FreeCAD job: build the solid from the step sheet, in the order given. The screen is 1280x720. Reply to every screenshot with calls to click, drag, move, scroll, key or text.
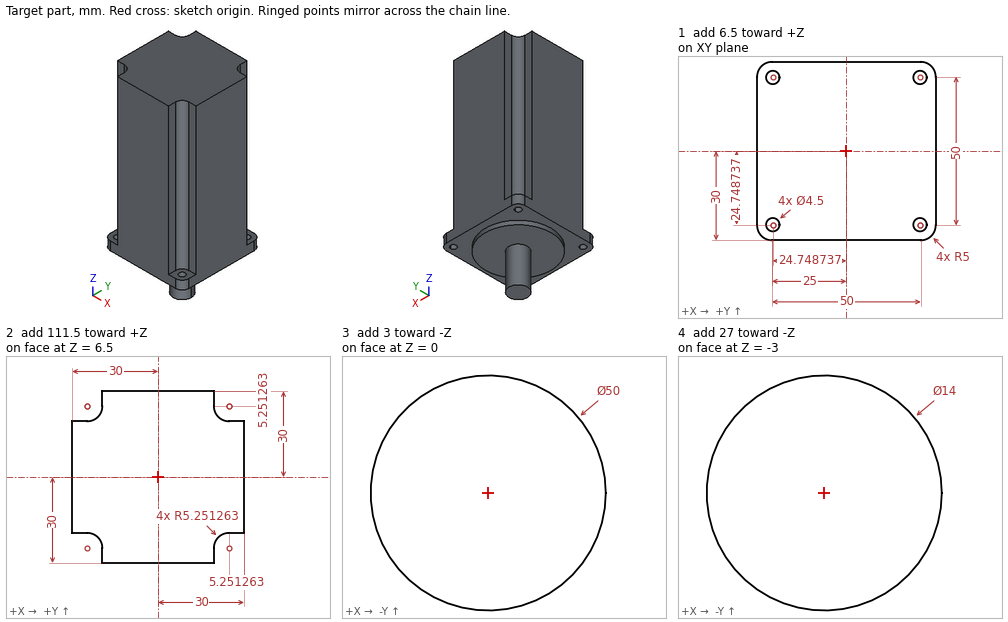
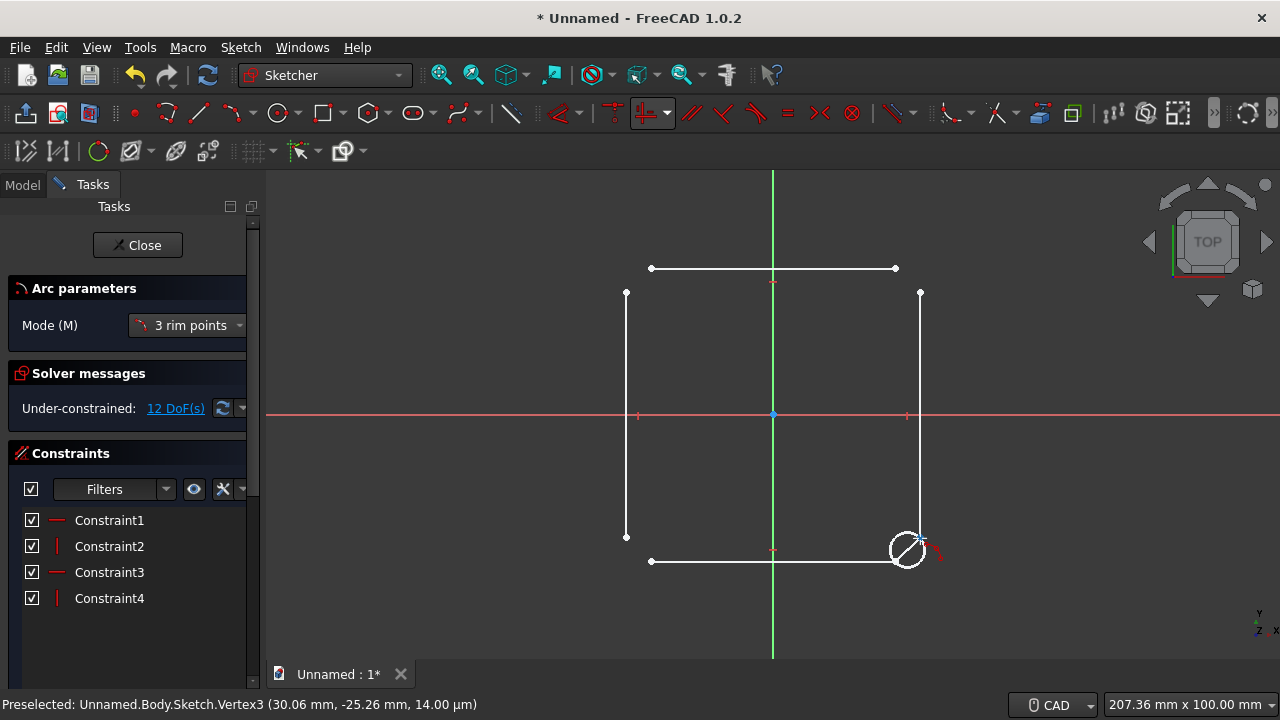
scroll(913, 554, up, 4)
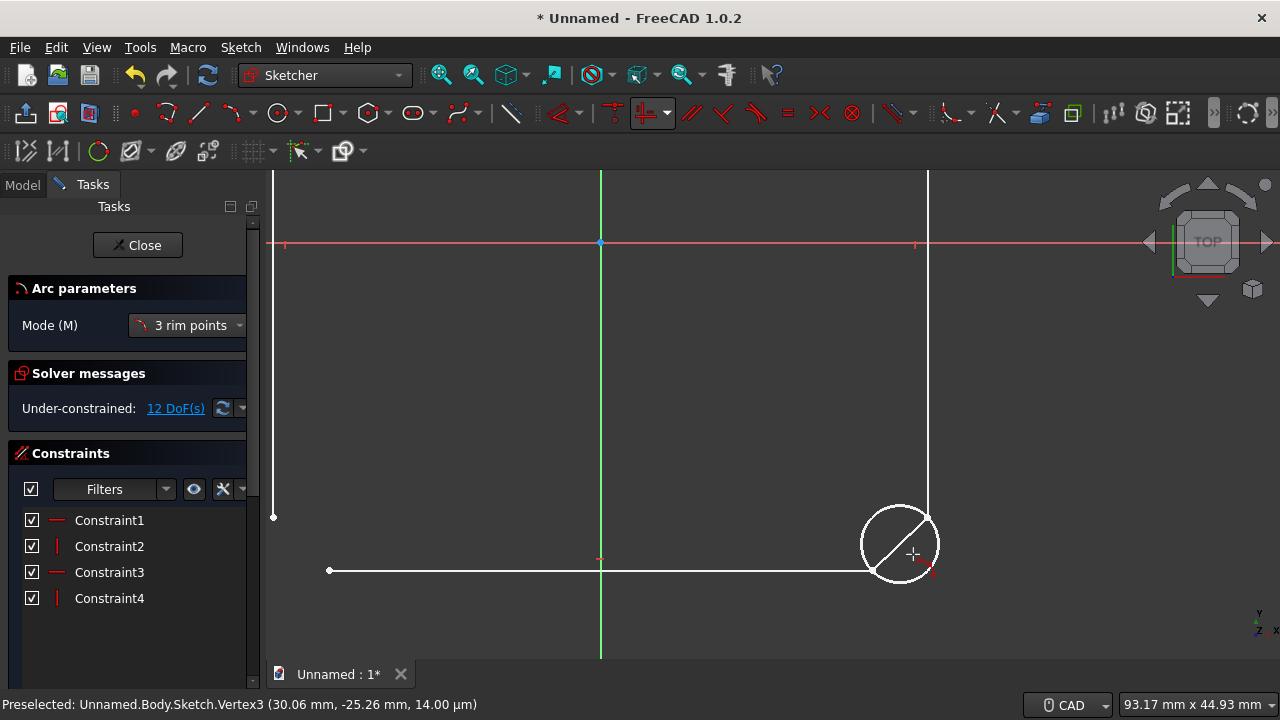
click(911, 553)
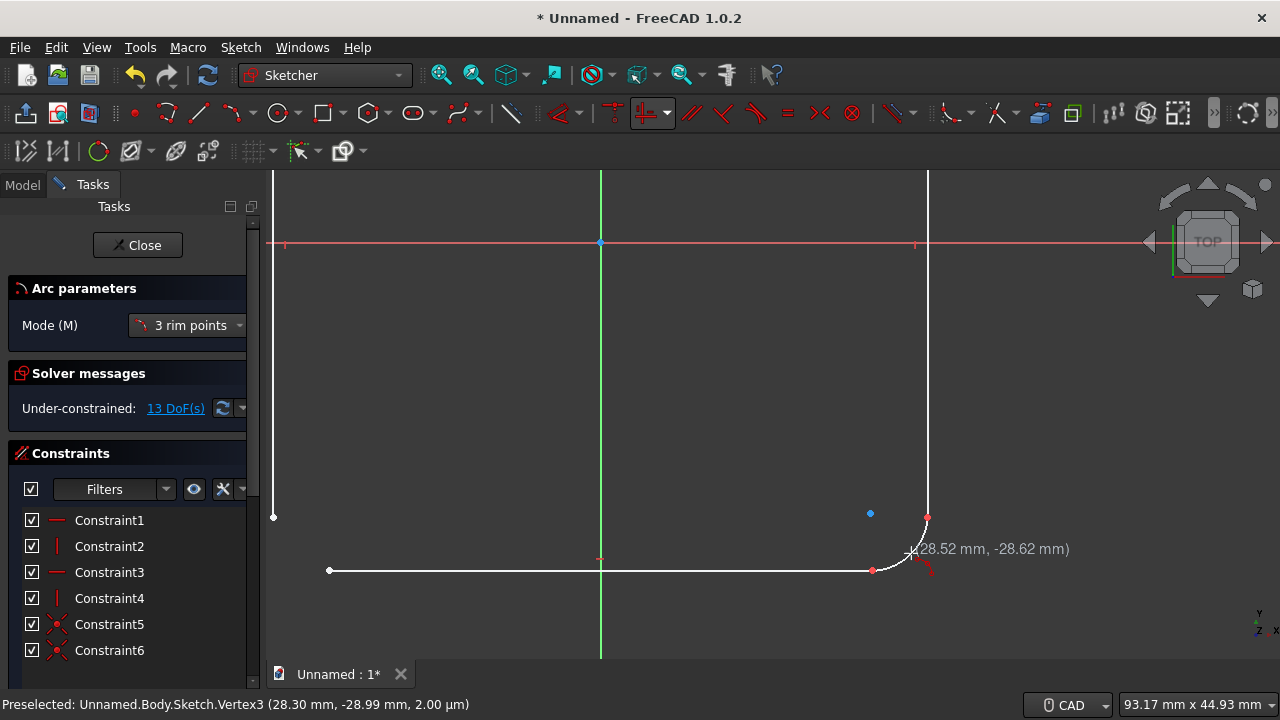
scroll(789, 555, down, 4)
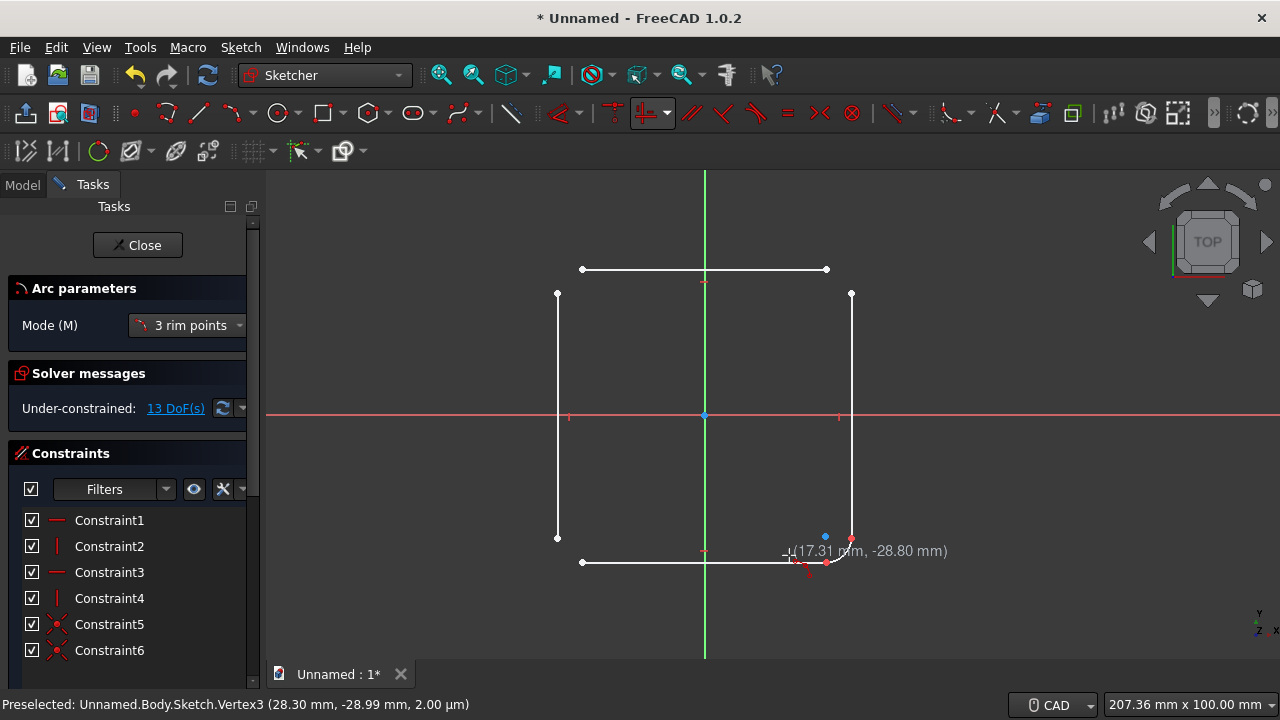
click(852, 294)
click(827, 270)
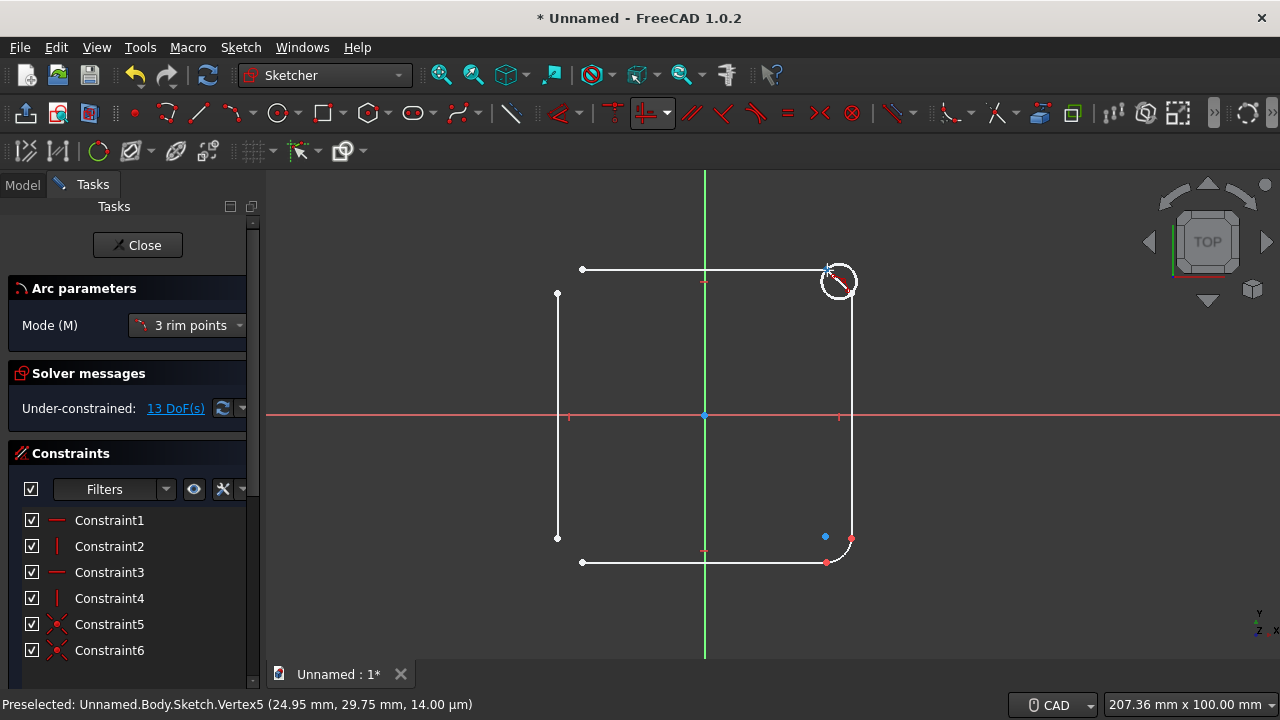
scroll(844, 276, up, 4)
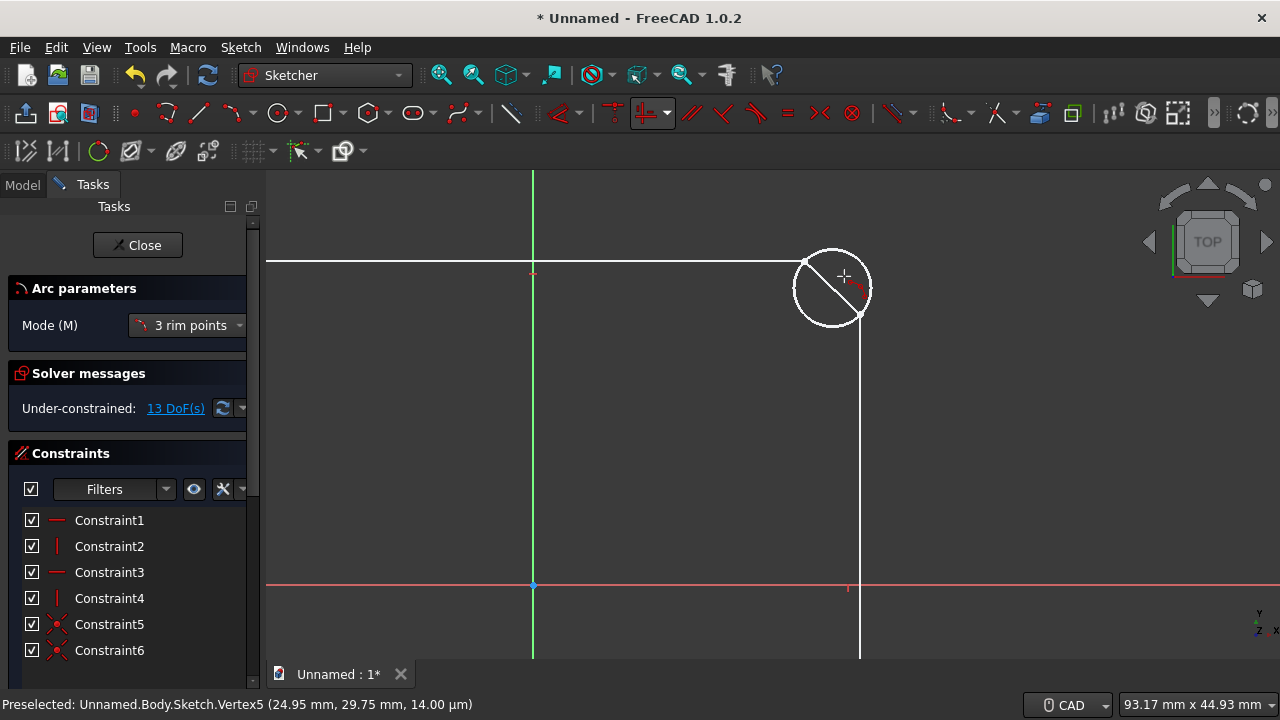
click(844, 275)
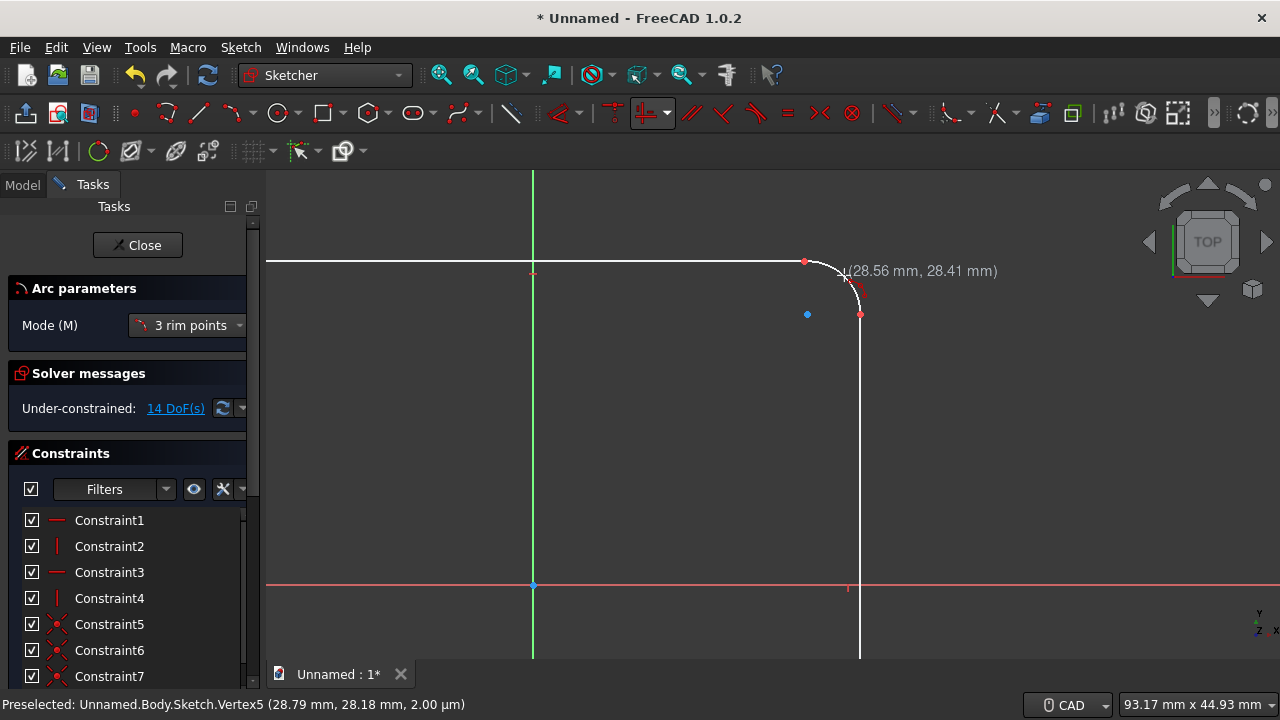
scroll(844, 275, down, 4)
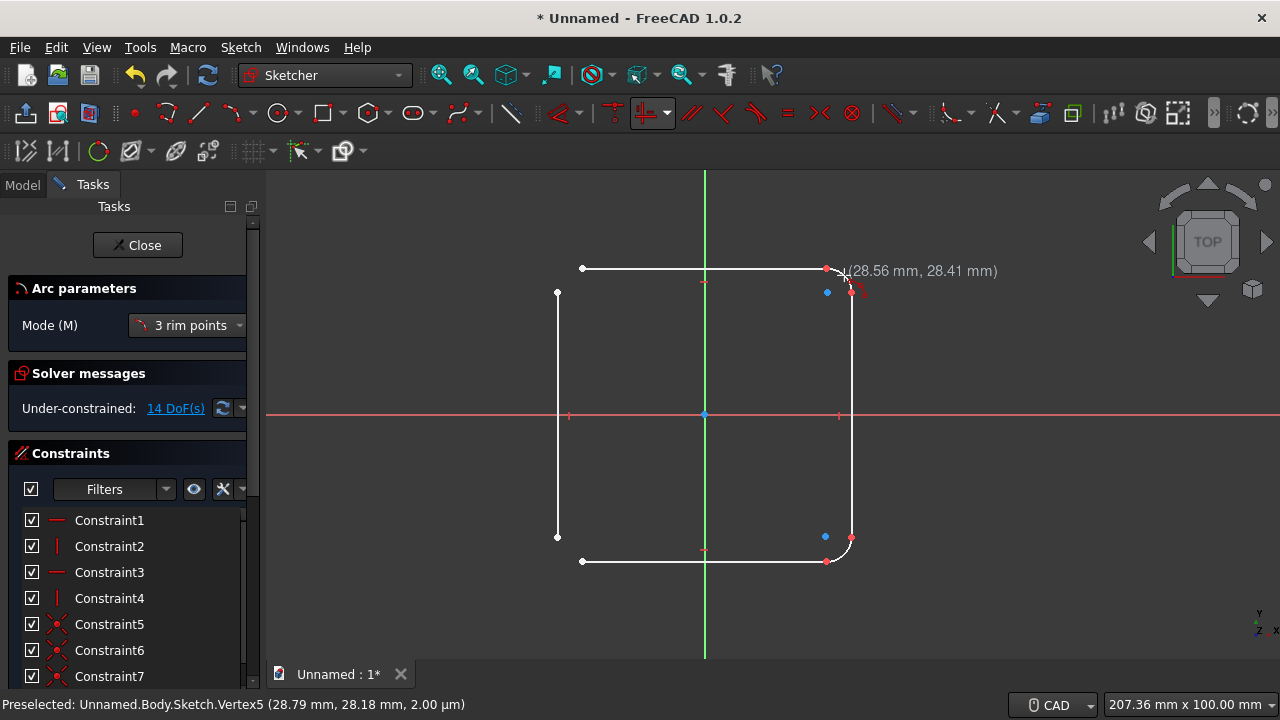
click(583, 269)
click(558, 293)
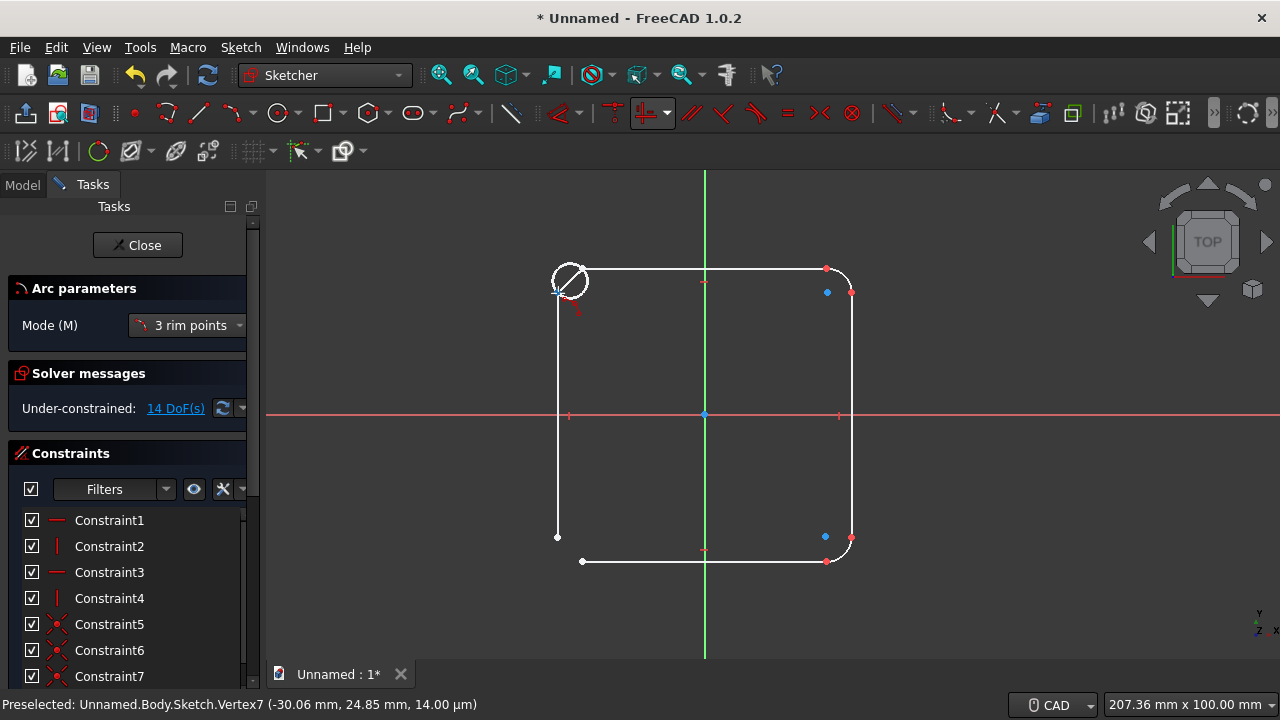
scroll(565, 275, up, 4)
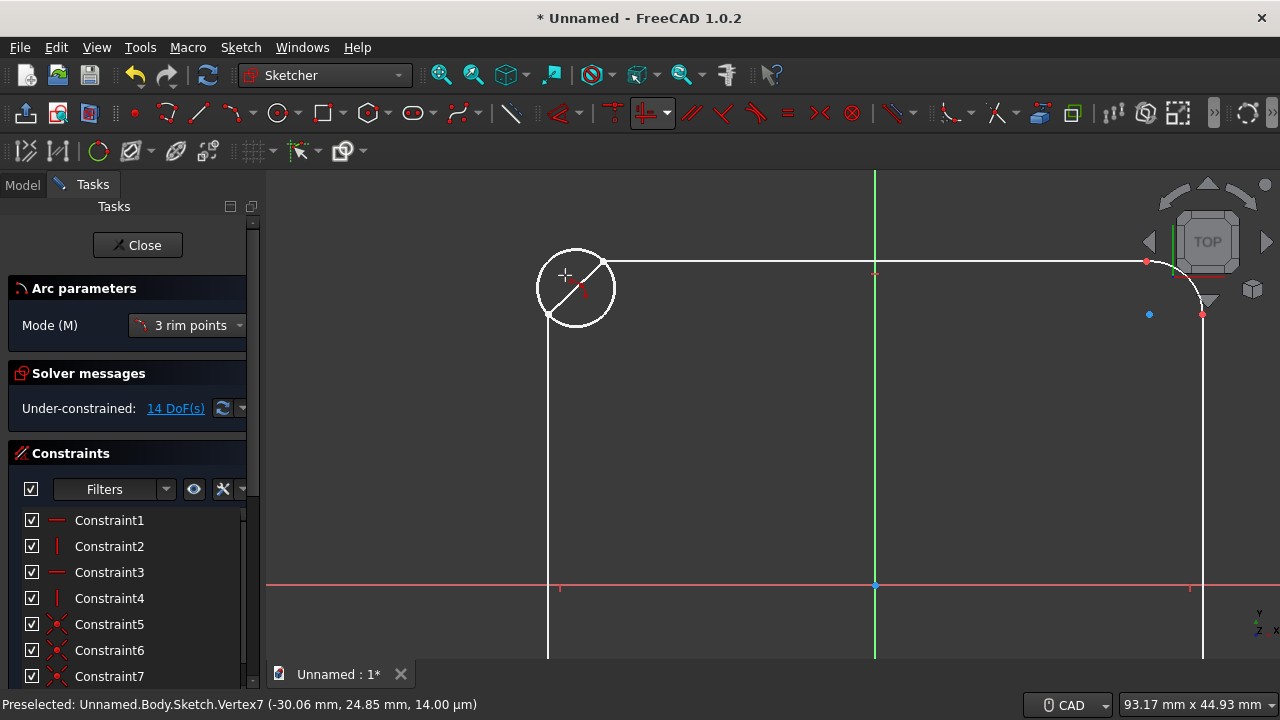
click(565, 275)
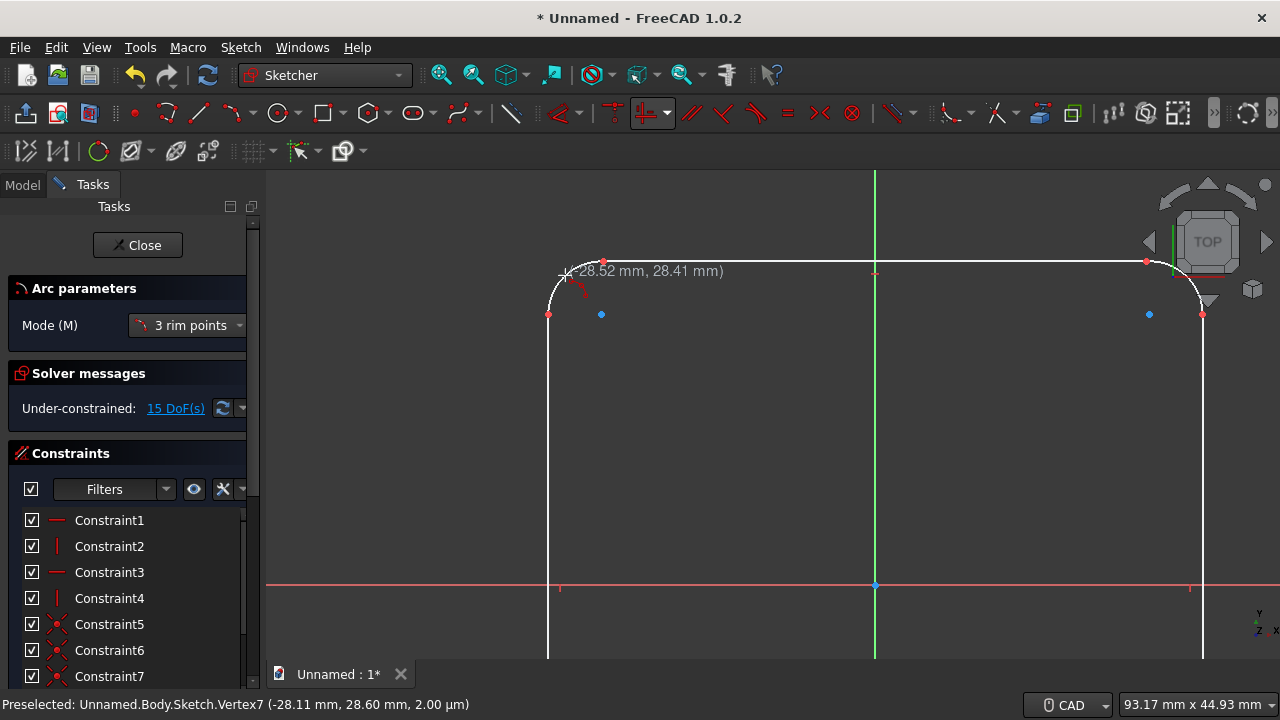
scroll(565, 275, down, 4)